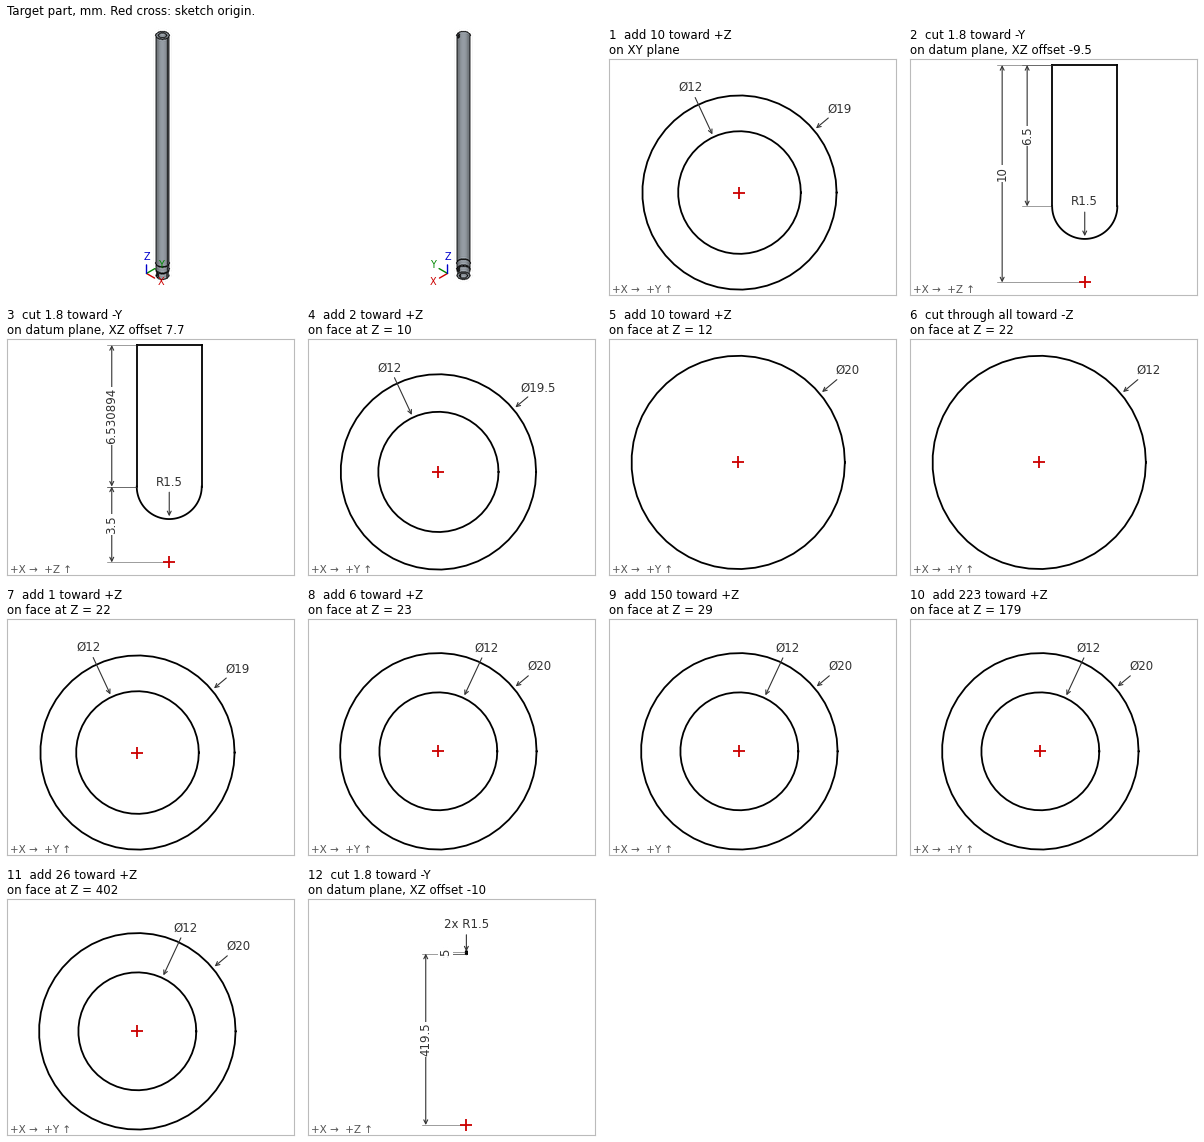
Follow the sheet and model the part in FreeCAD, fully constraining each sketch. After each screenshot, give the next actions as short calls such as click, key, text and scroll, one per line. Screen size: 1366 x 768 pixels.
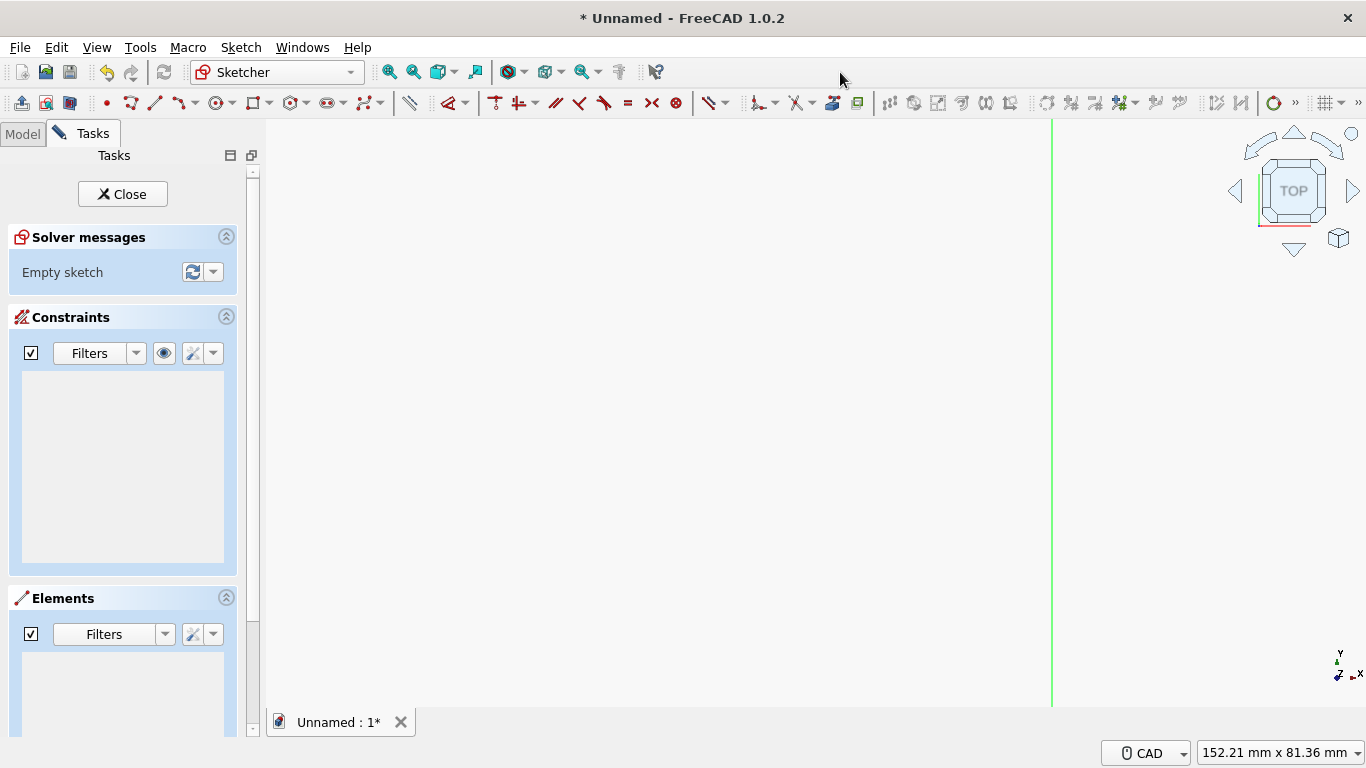
scroll(748, 413, down, 5)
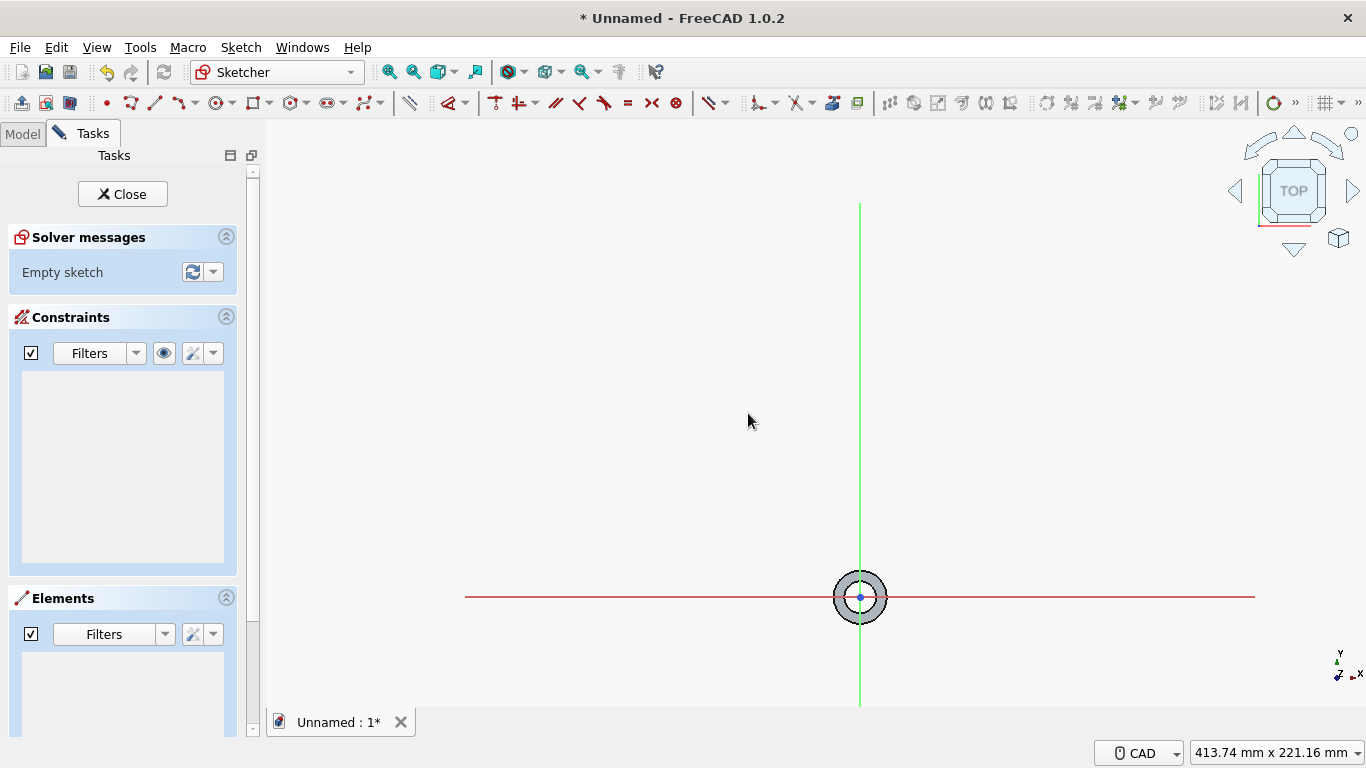
scroll(878, 626, up, 10)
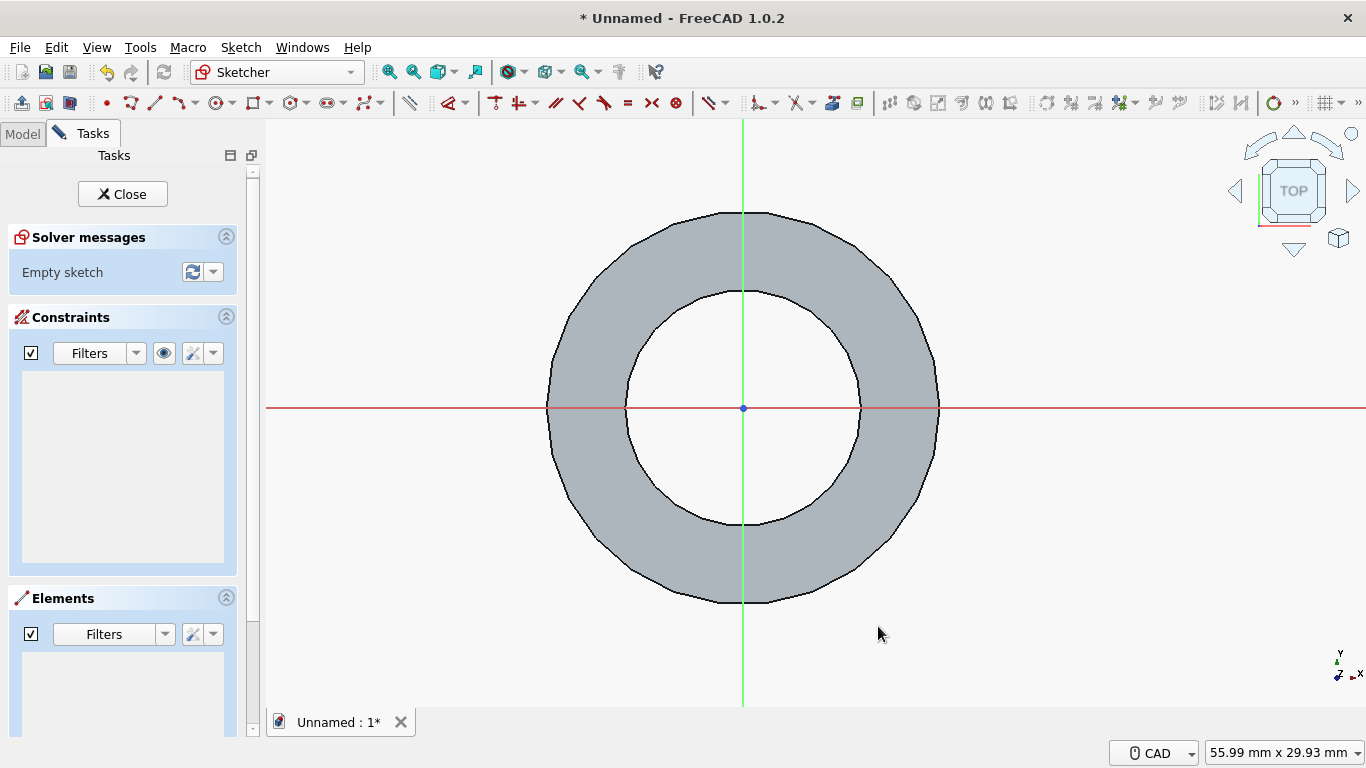
click(216, 104)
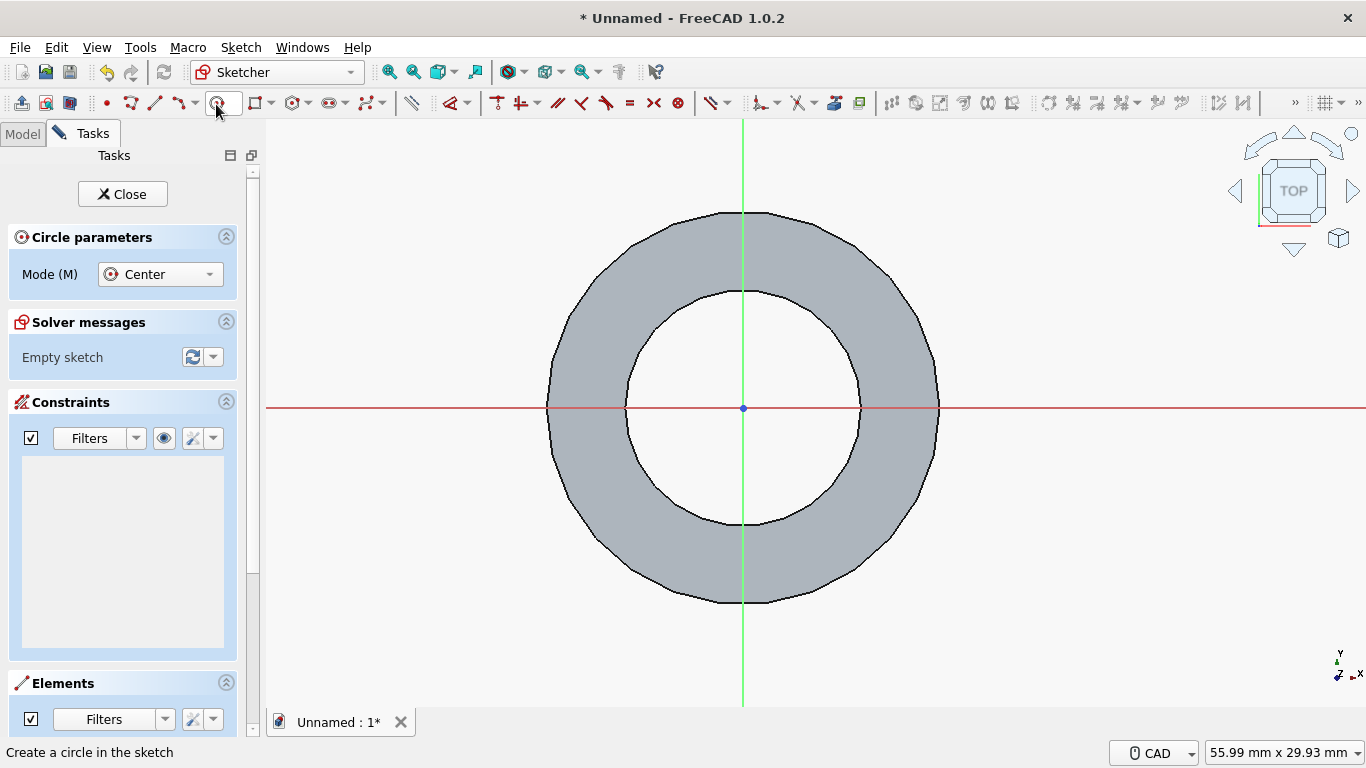
click(743, 408)
click(882, 269)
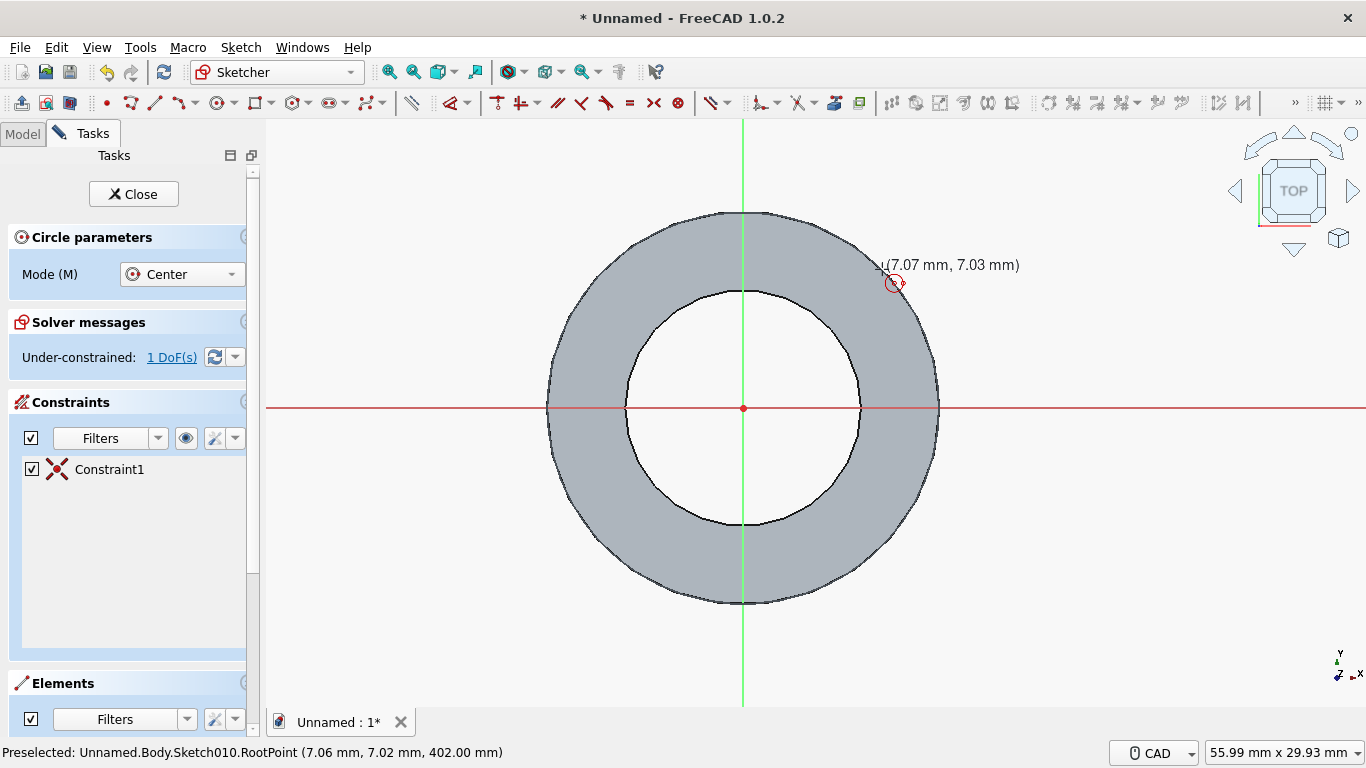
click(743, 408)
click(826, 325)
key(Escape)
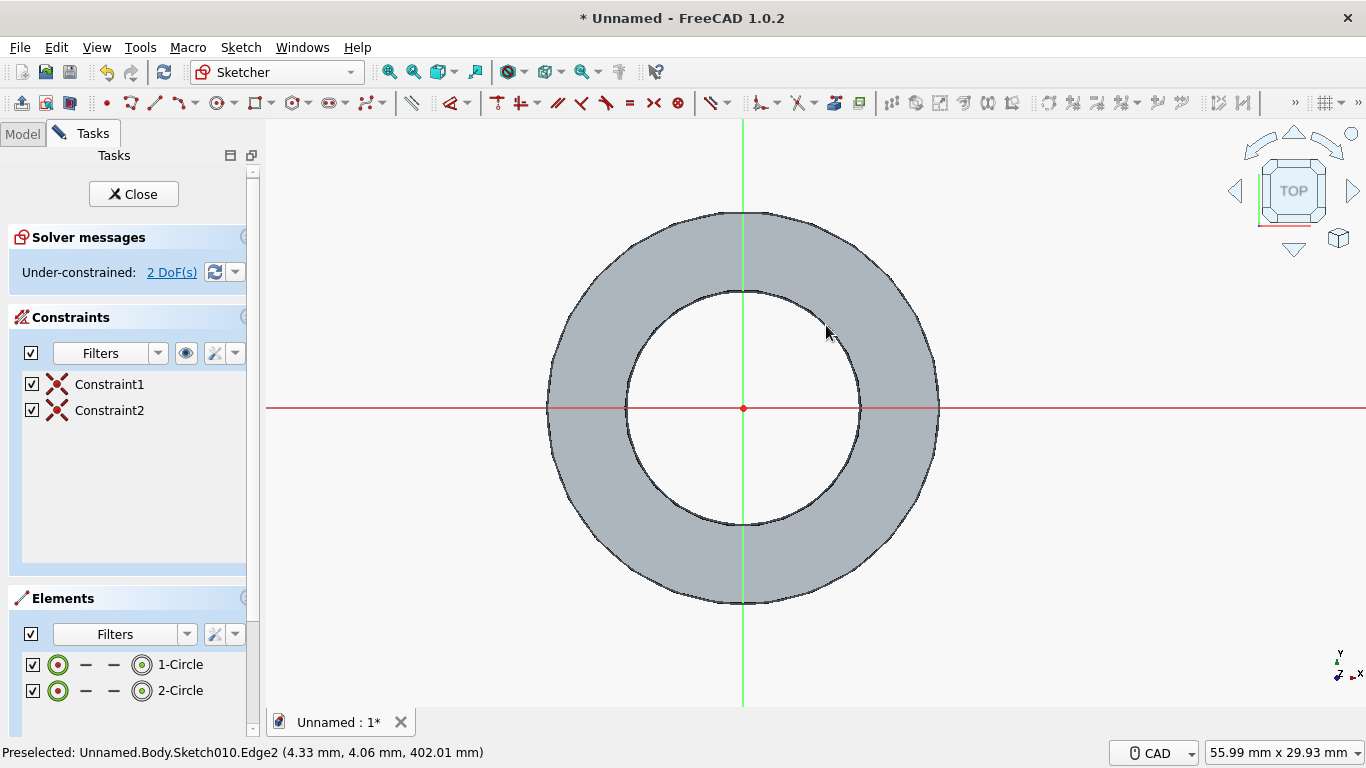
click(450, 104)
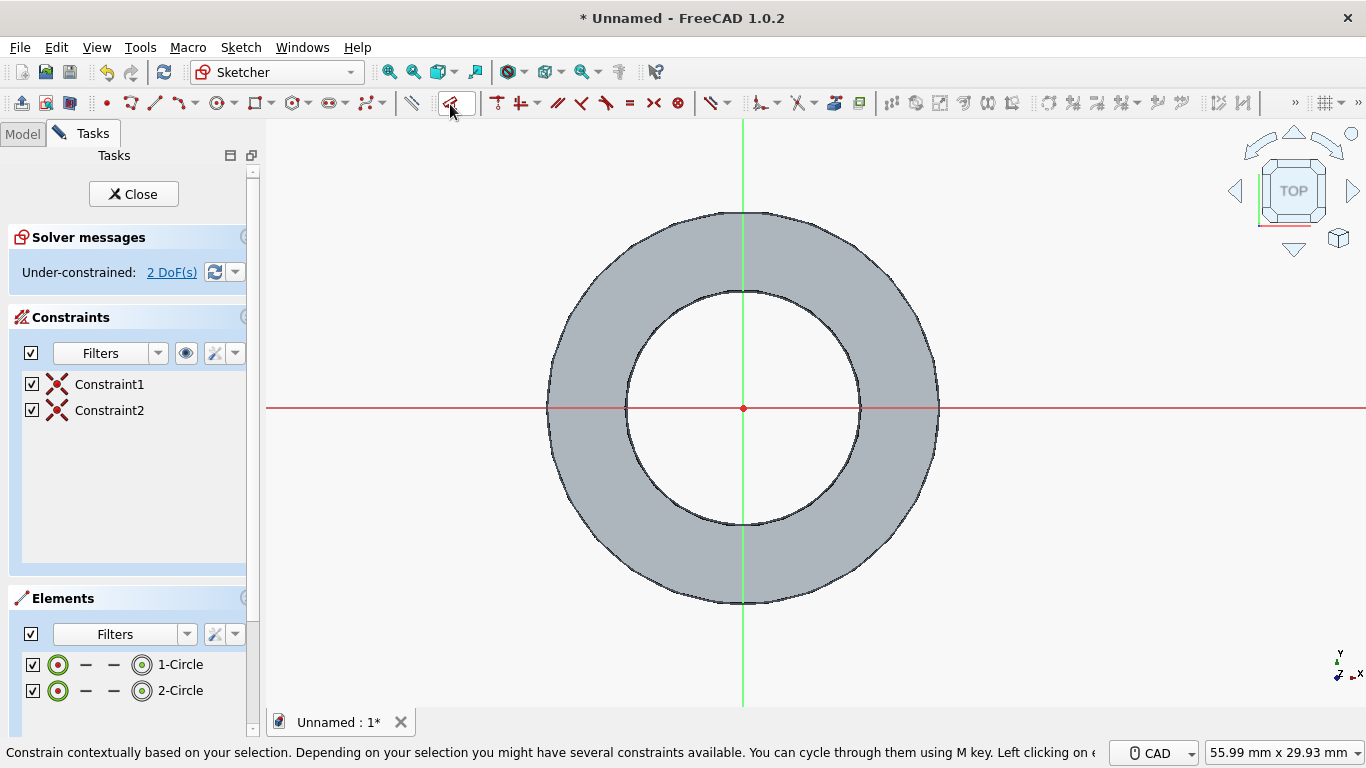
click(881, 269)
click(904, 246)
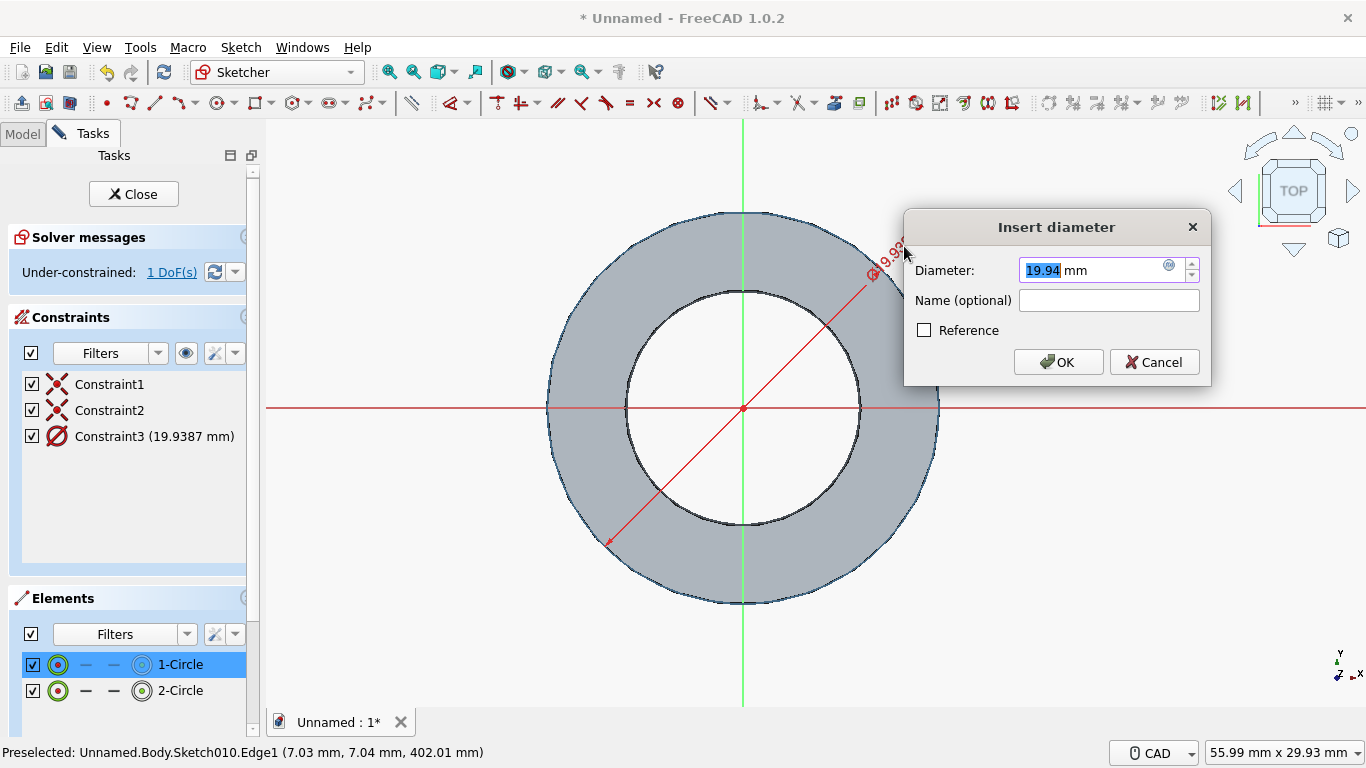
text(20)
key(Return)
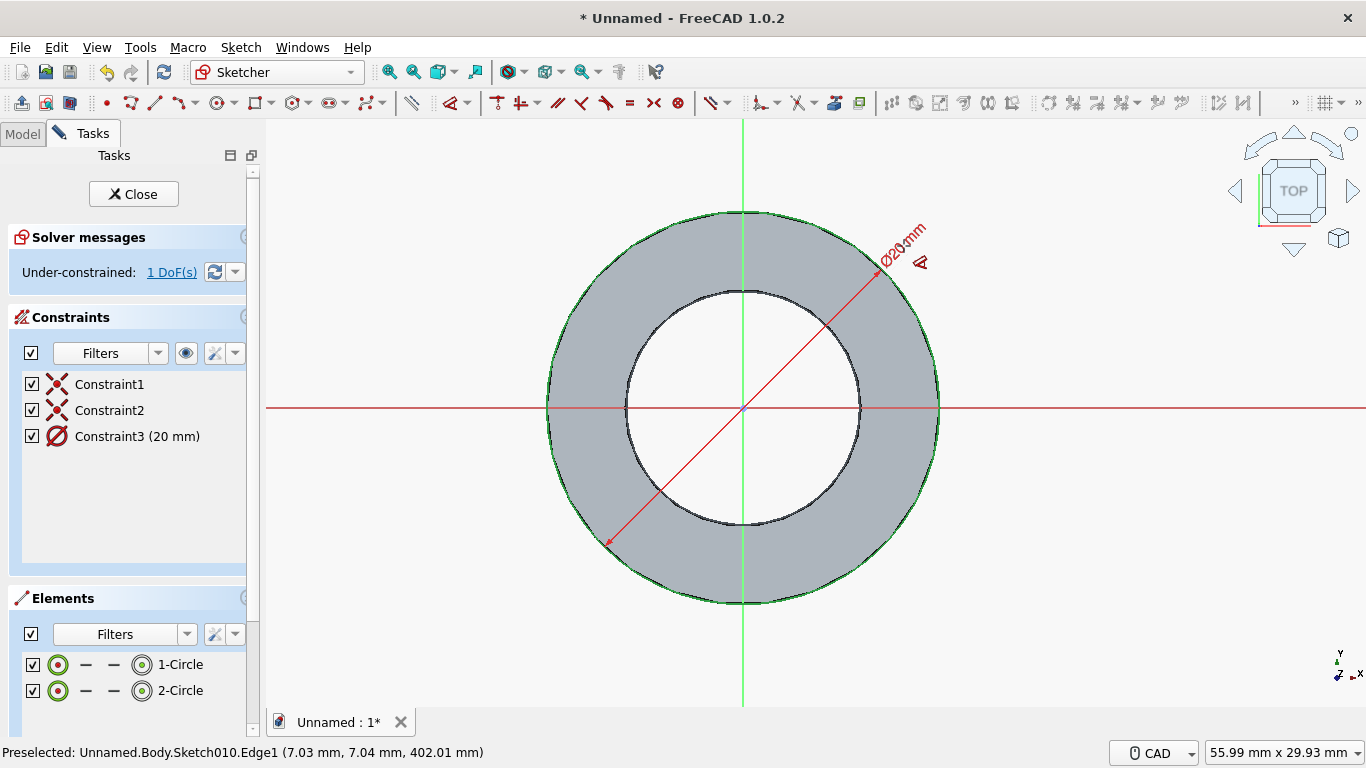
click(825, 325)
click(847, 302)